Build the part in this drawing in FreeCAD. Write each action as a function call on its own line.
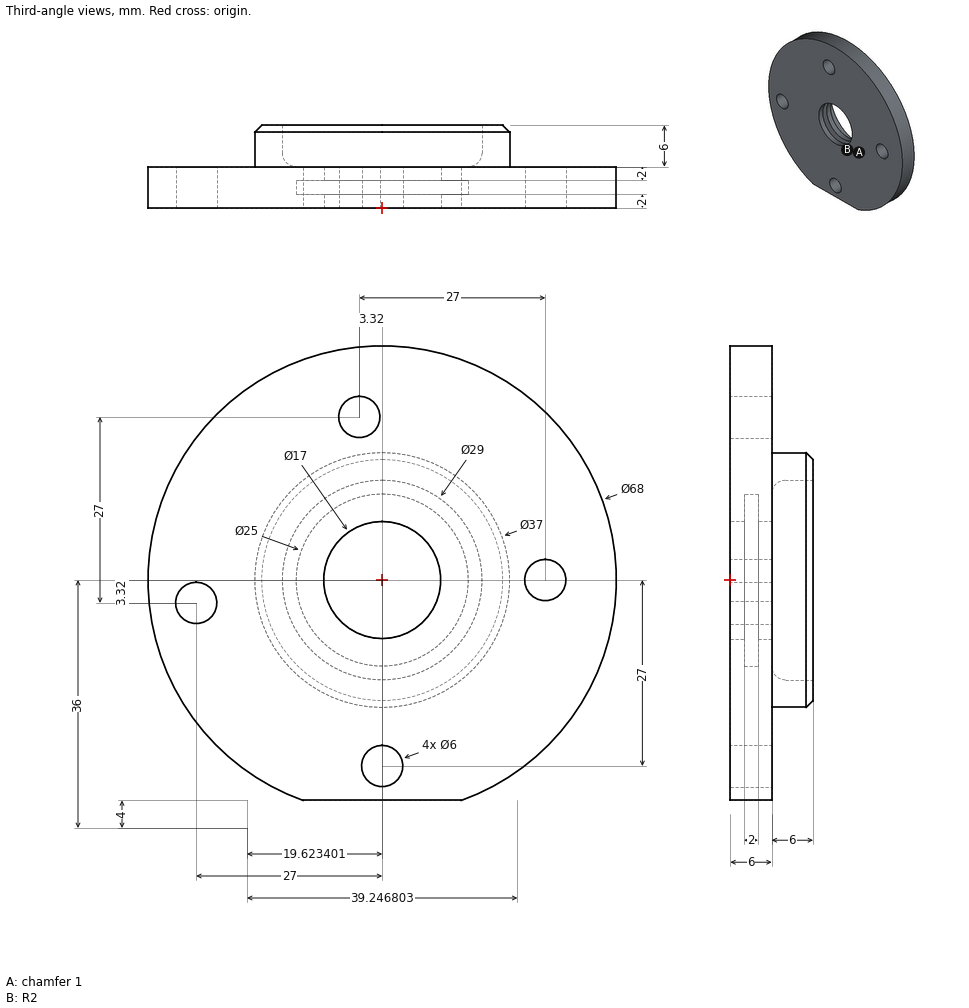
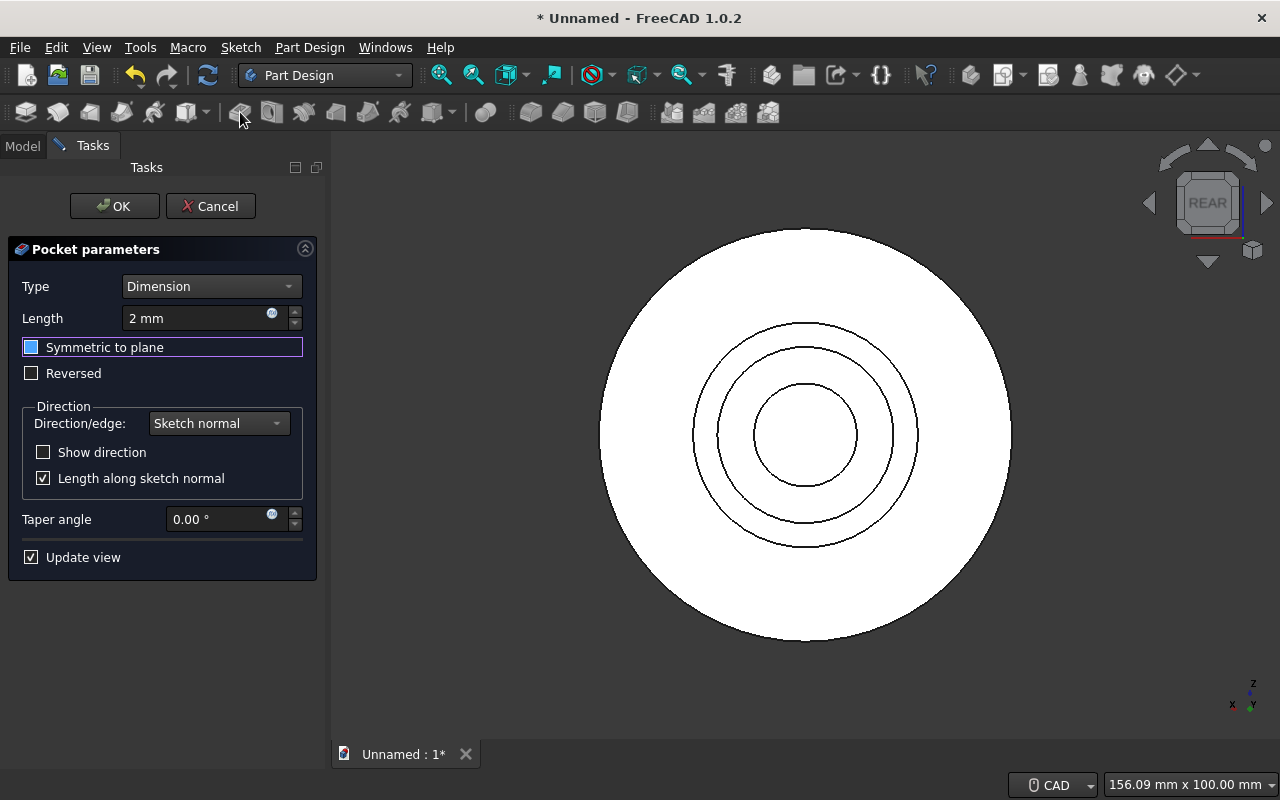
click(115, 206)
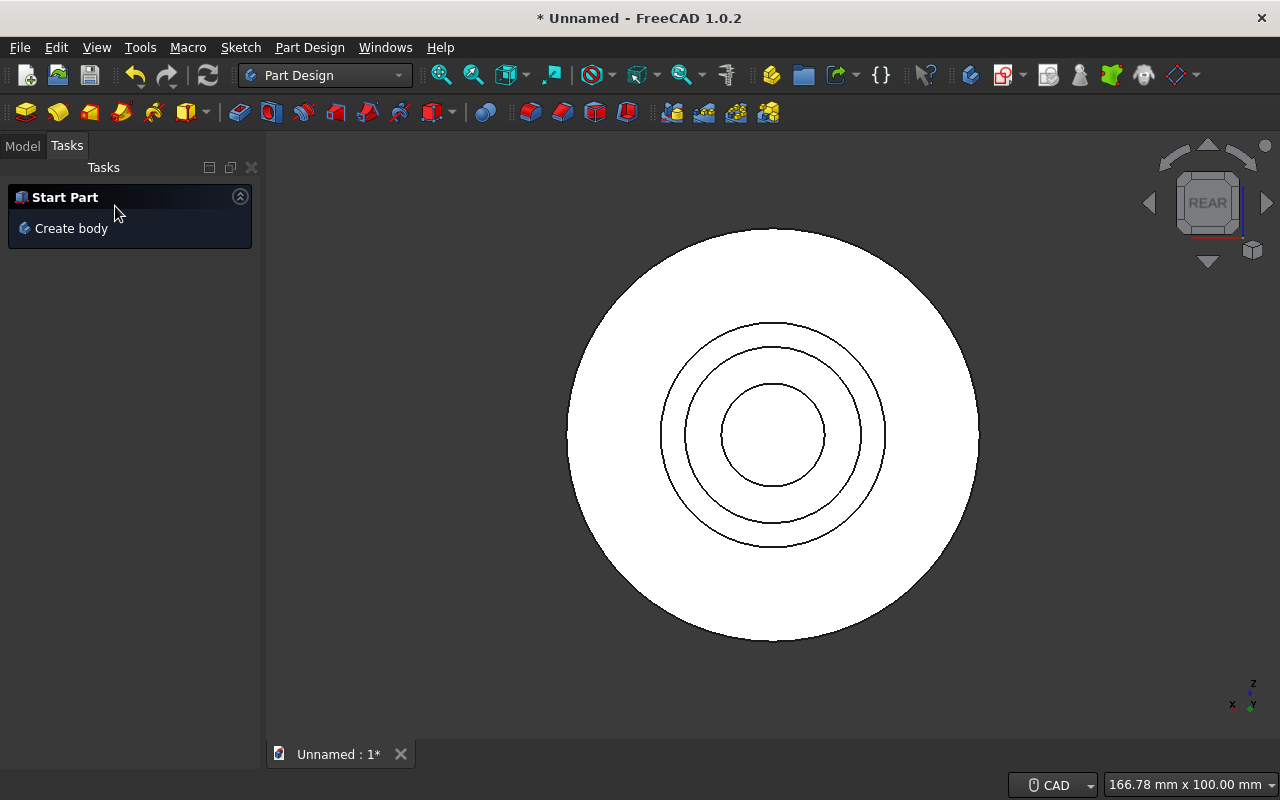
click(773, 434)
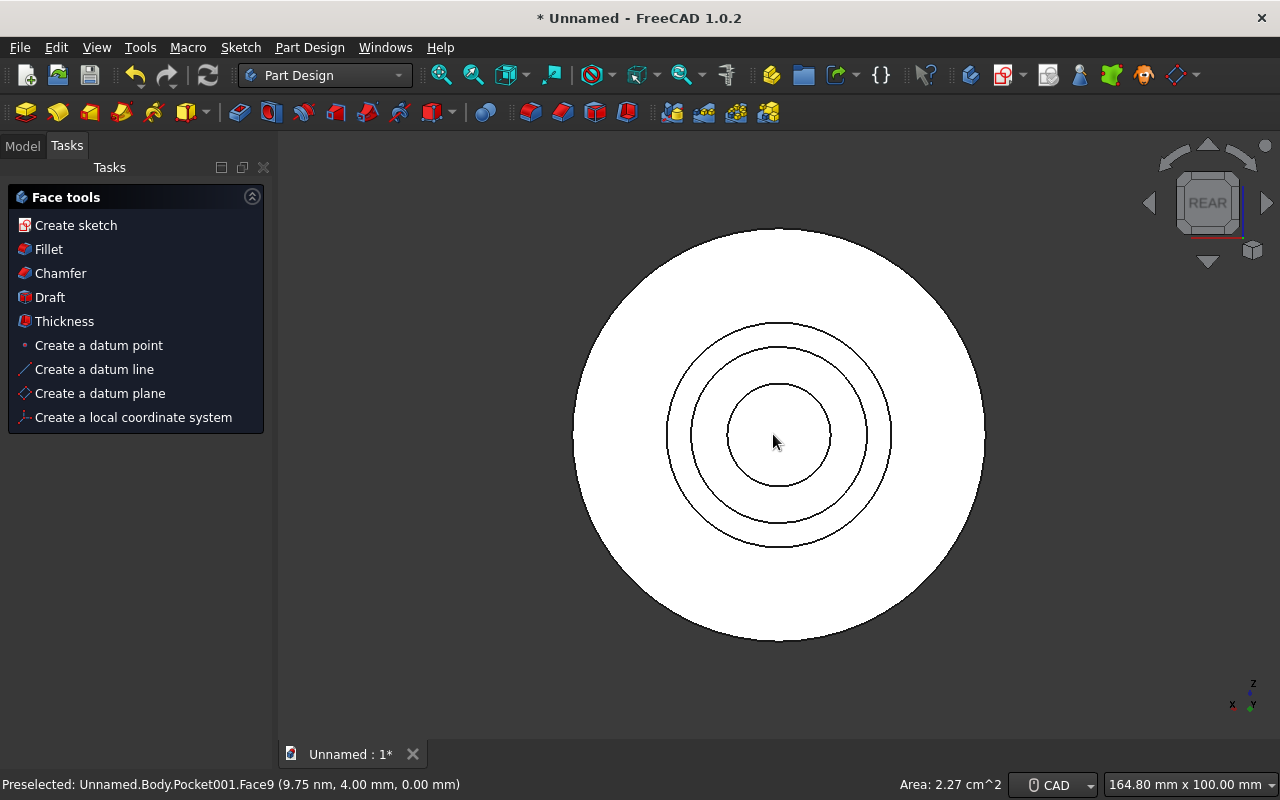
click(1004, 76)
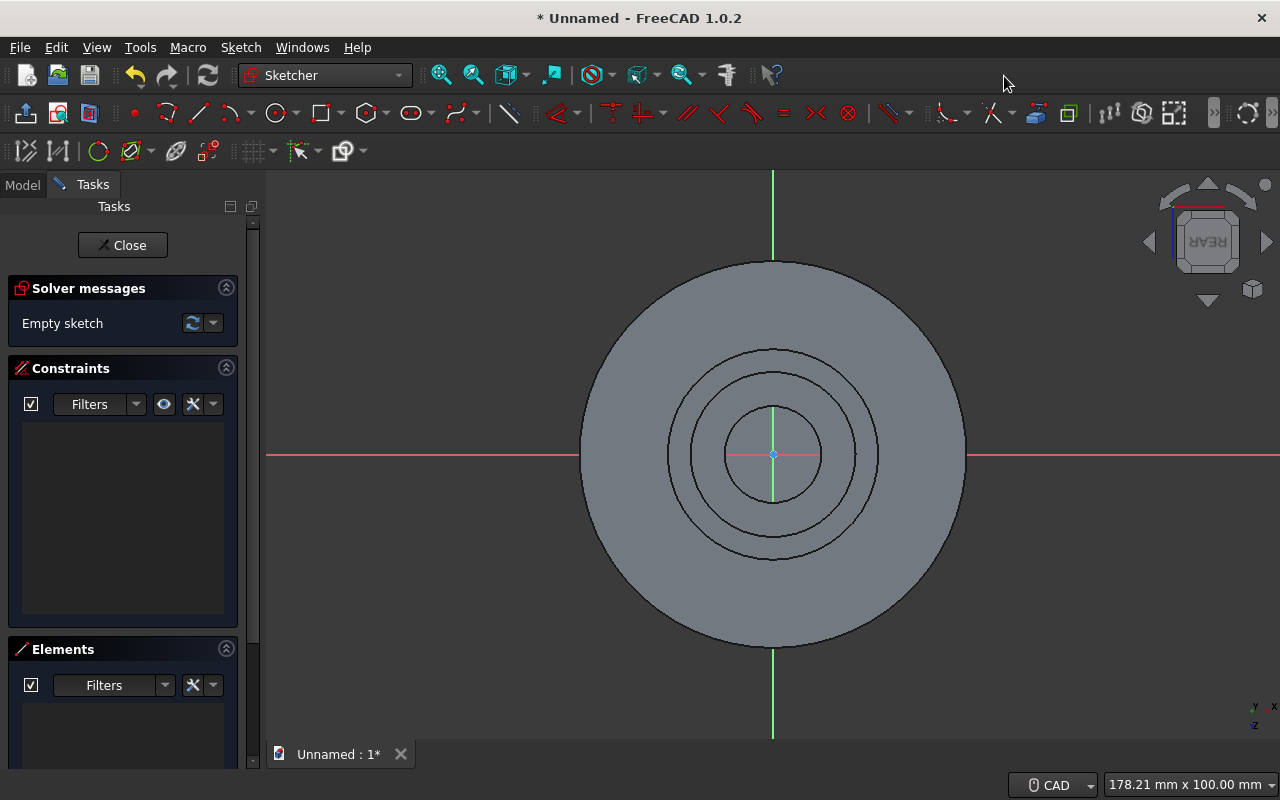
click(90, 114)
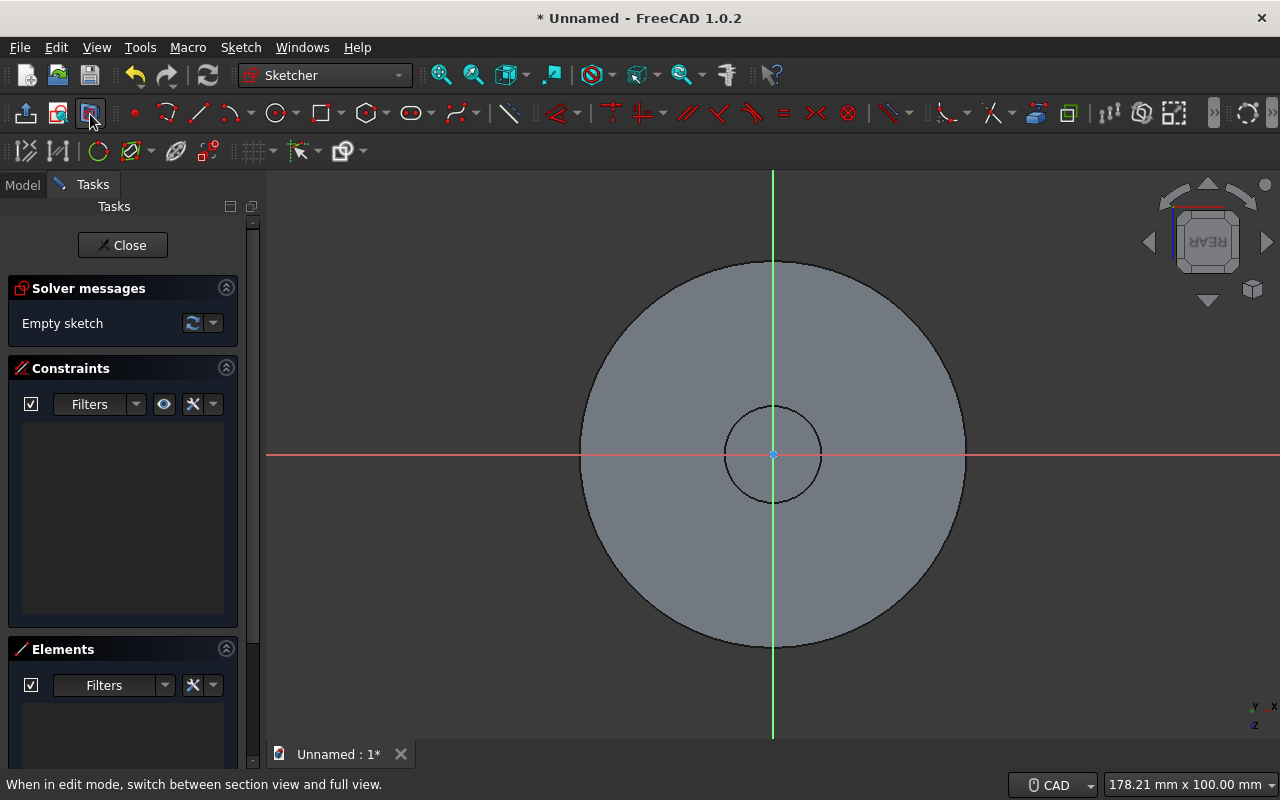
scroll(813, 454, up, 5)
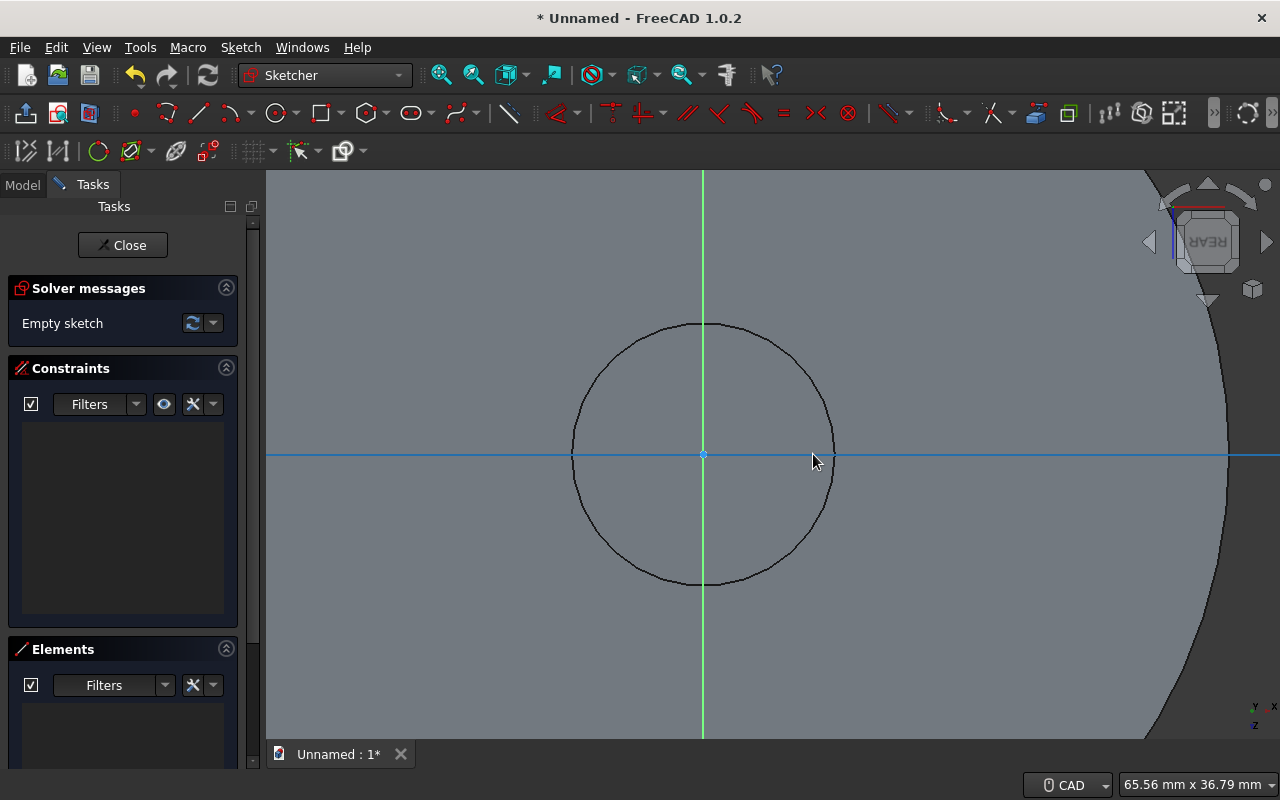
click(276, 114)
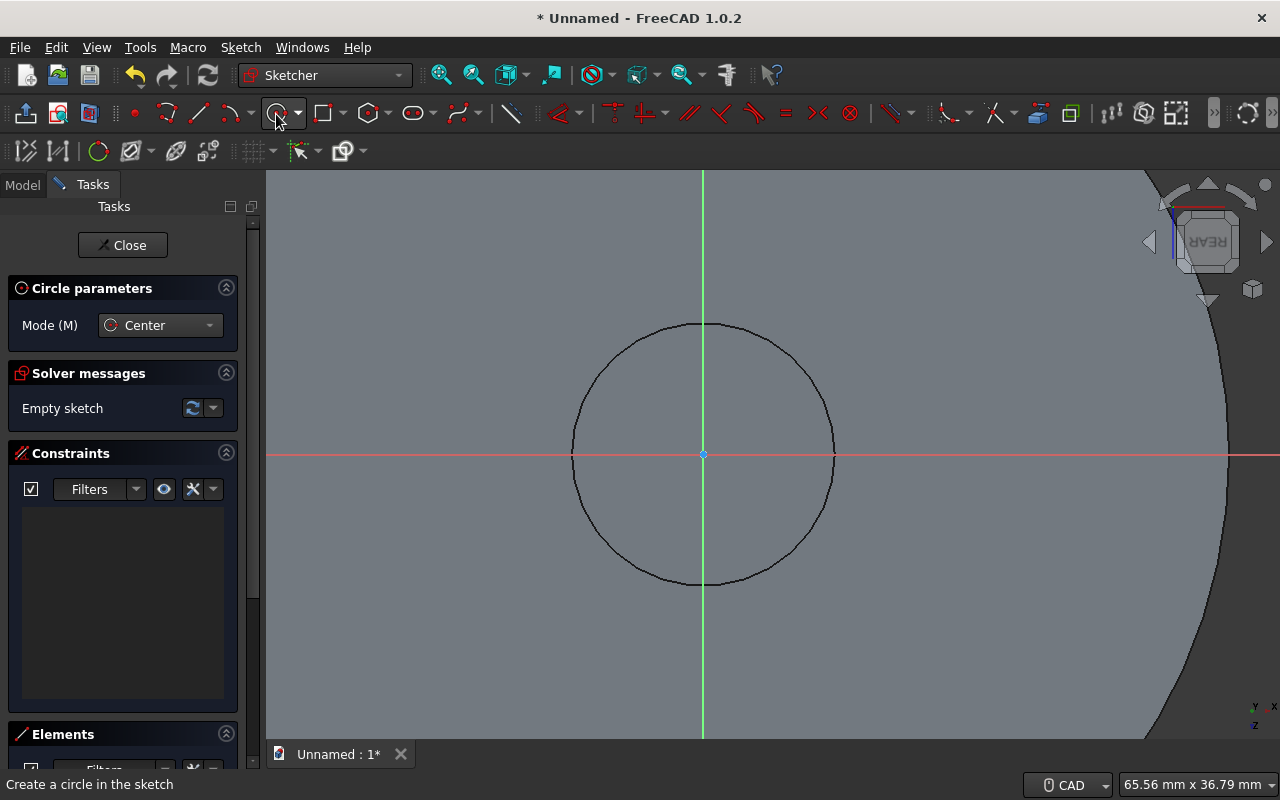
click(703, 454)
click(840, 318)
key(Escape)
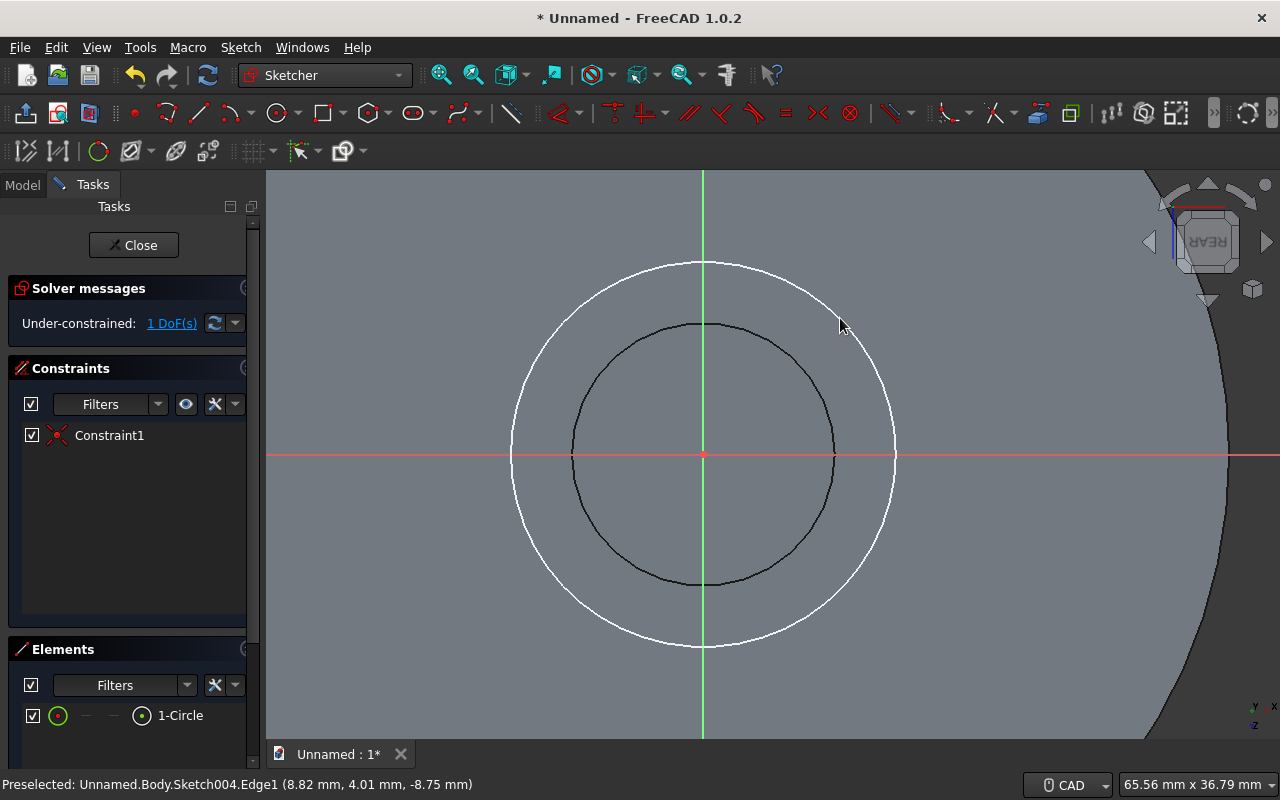
click(558, 114)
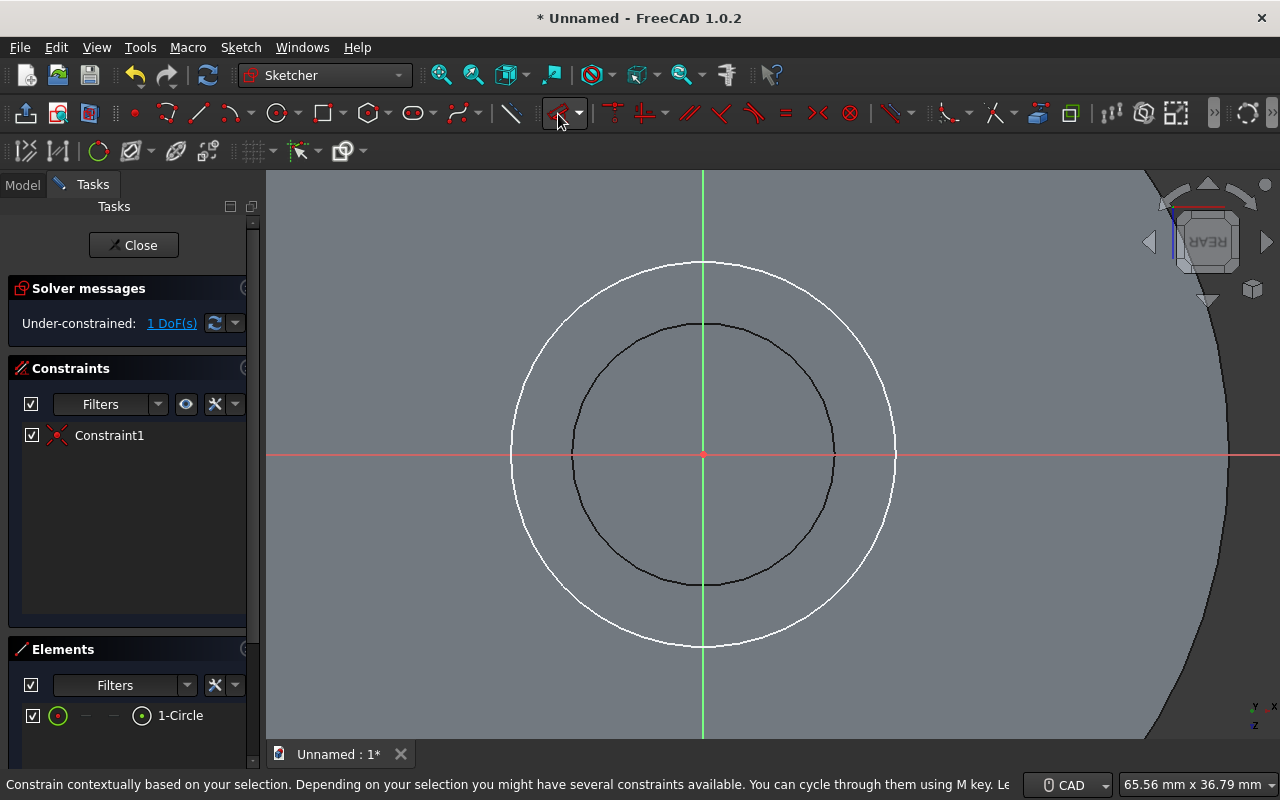
click(839, 318)
click(862, 295)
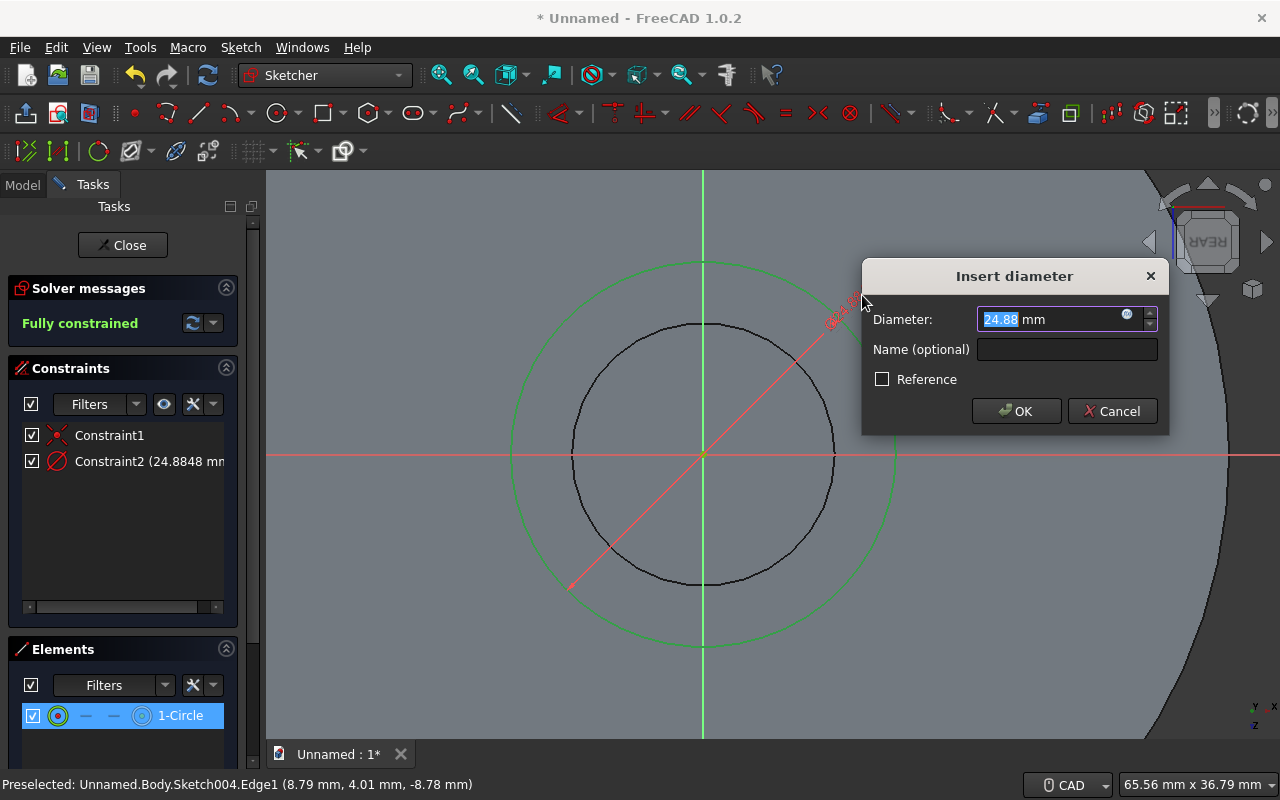
text(25)
key(Return)
key(Escape)